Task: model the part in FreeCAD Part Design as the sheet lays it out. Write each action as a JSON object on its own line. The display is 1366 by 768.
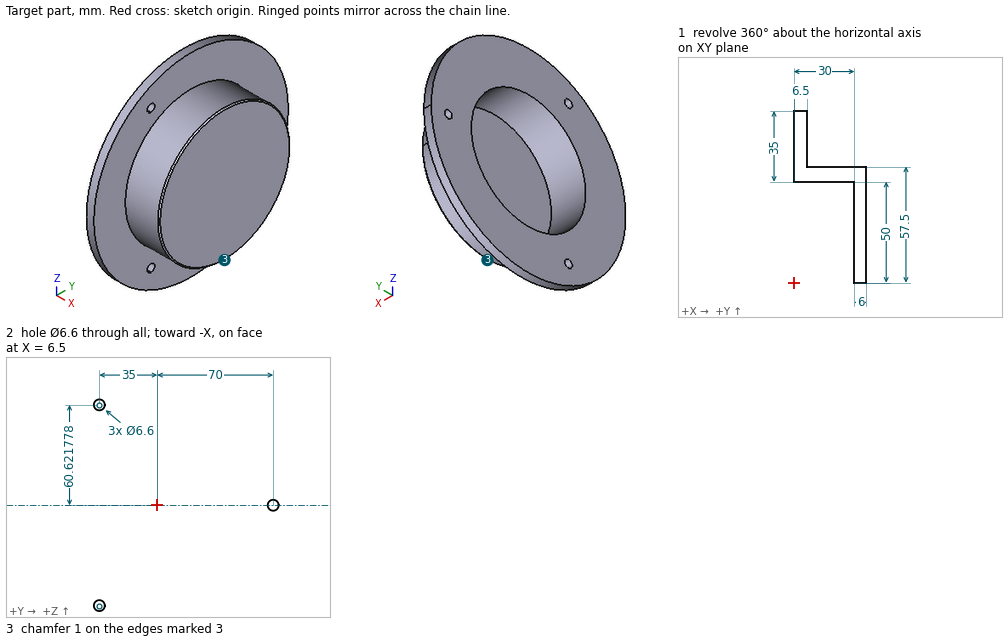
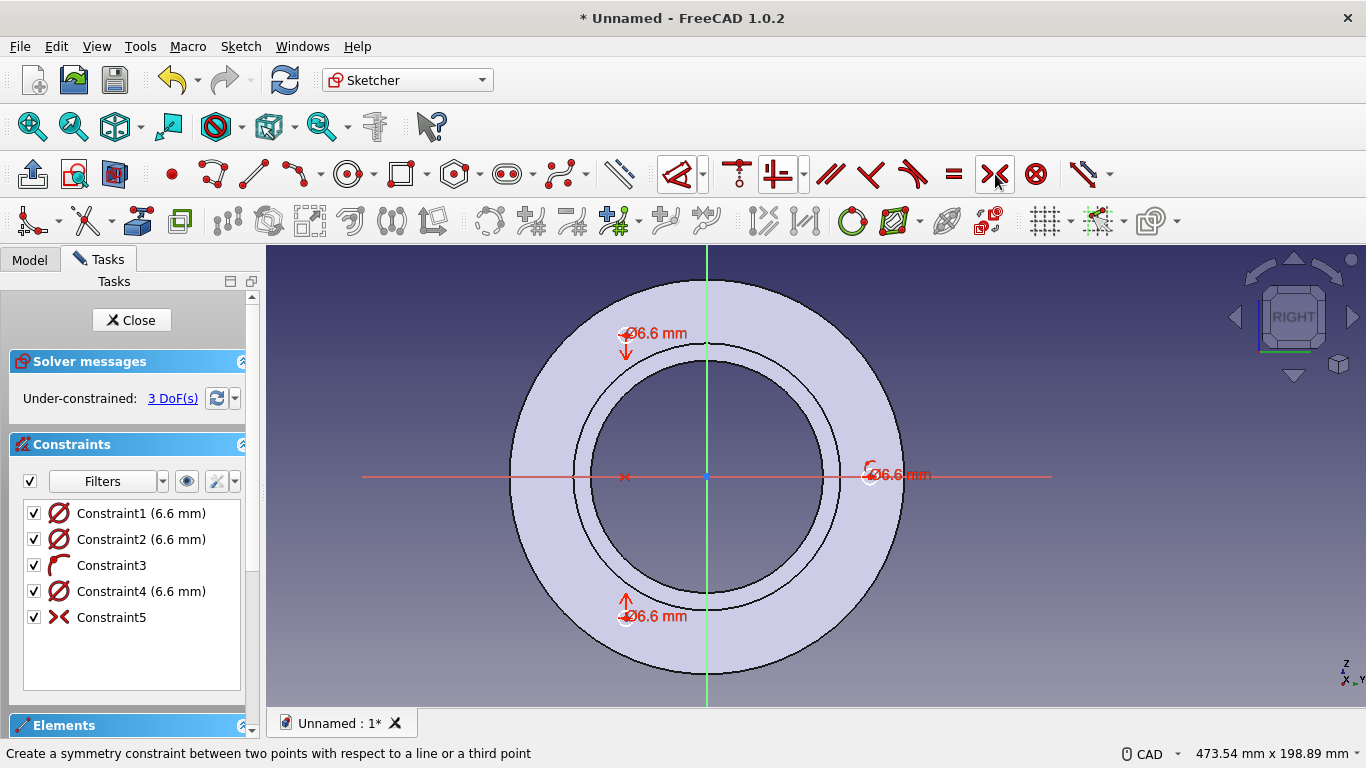
{"action": "left_click", "coordinate": [626, 335]}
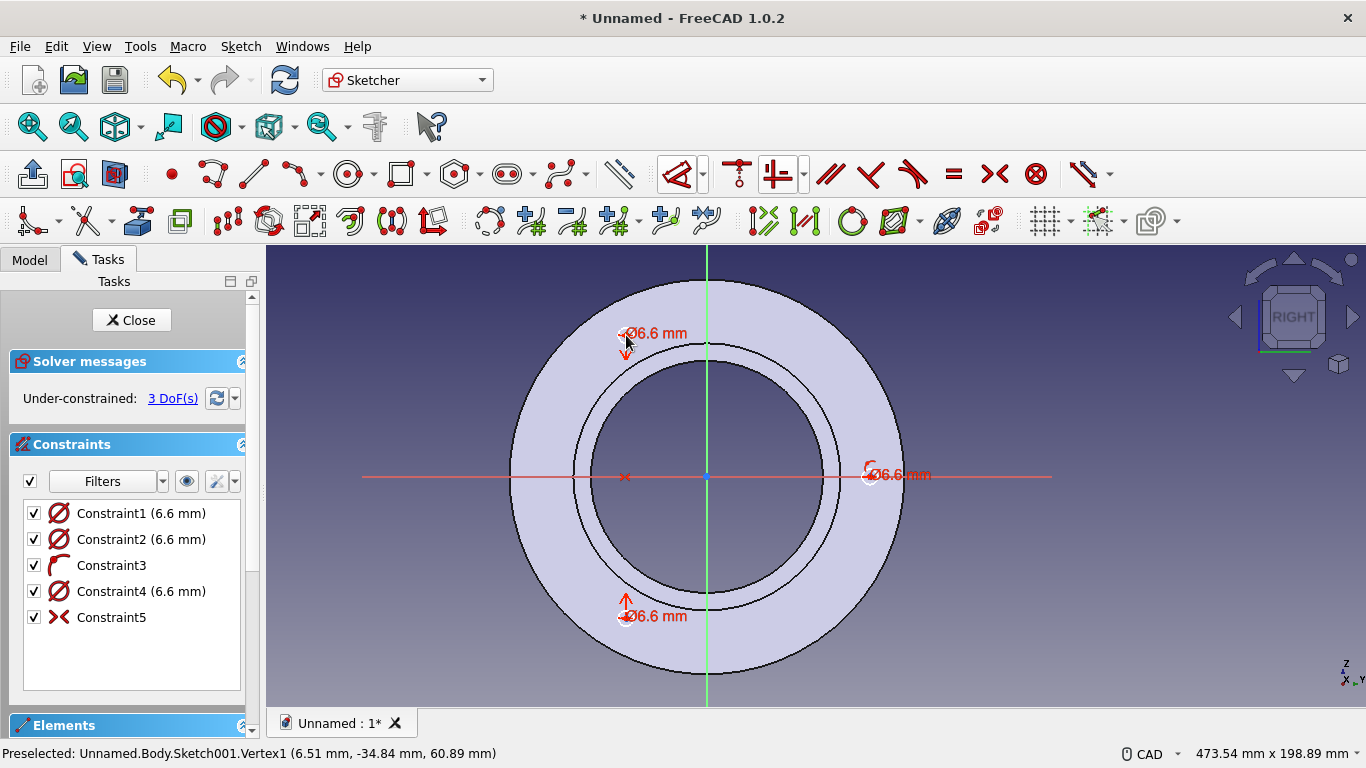
{"action": "left_click", "coordinate": [702, 174]}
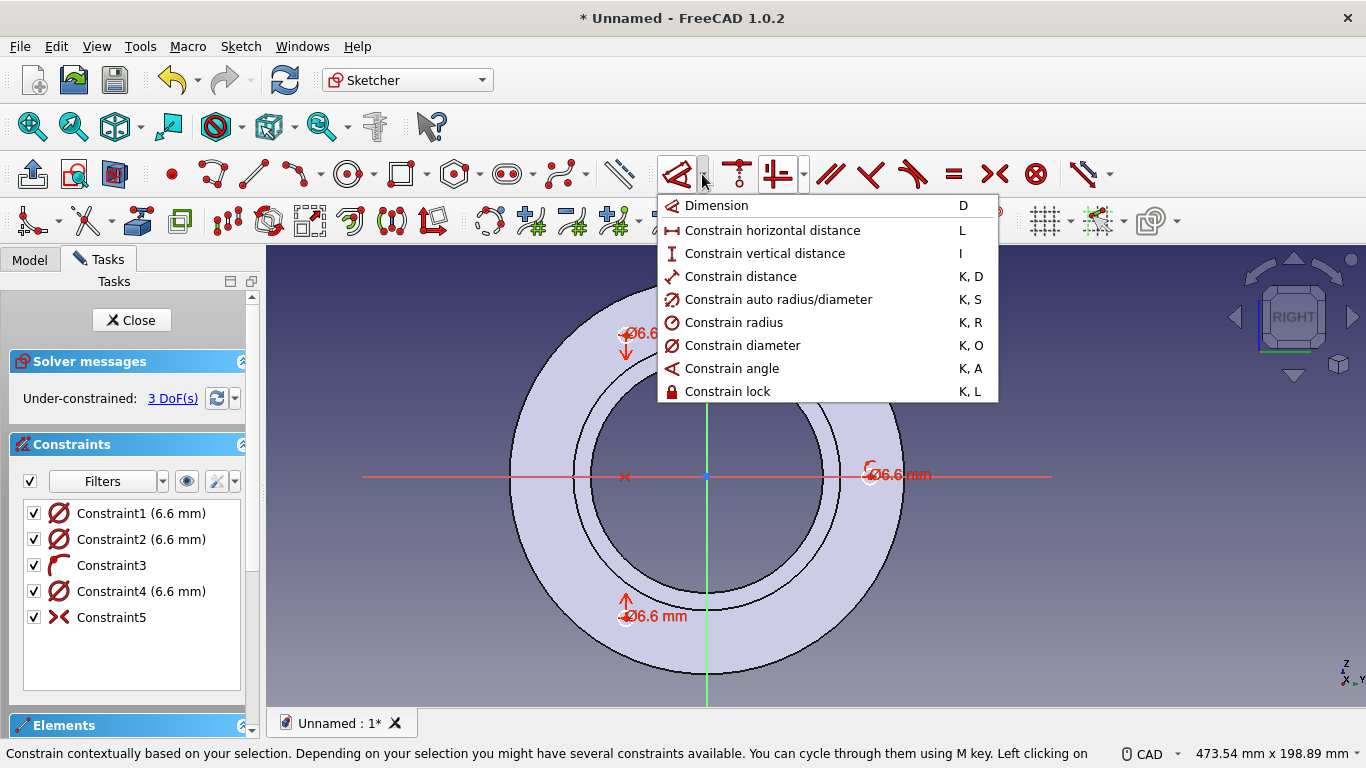
{"action": "left_click", "coordinate": [828, 230]}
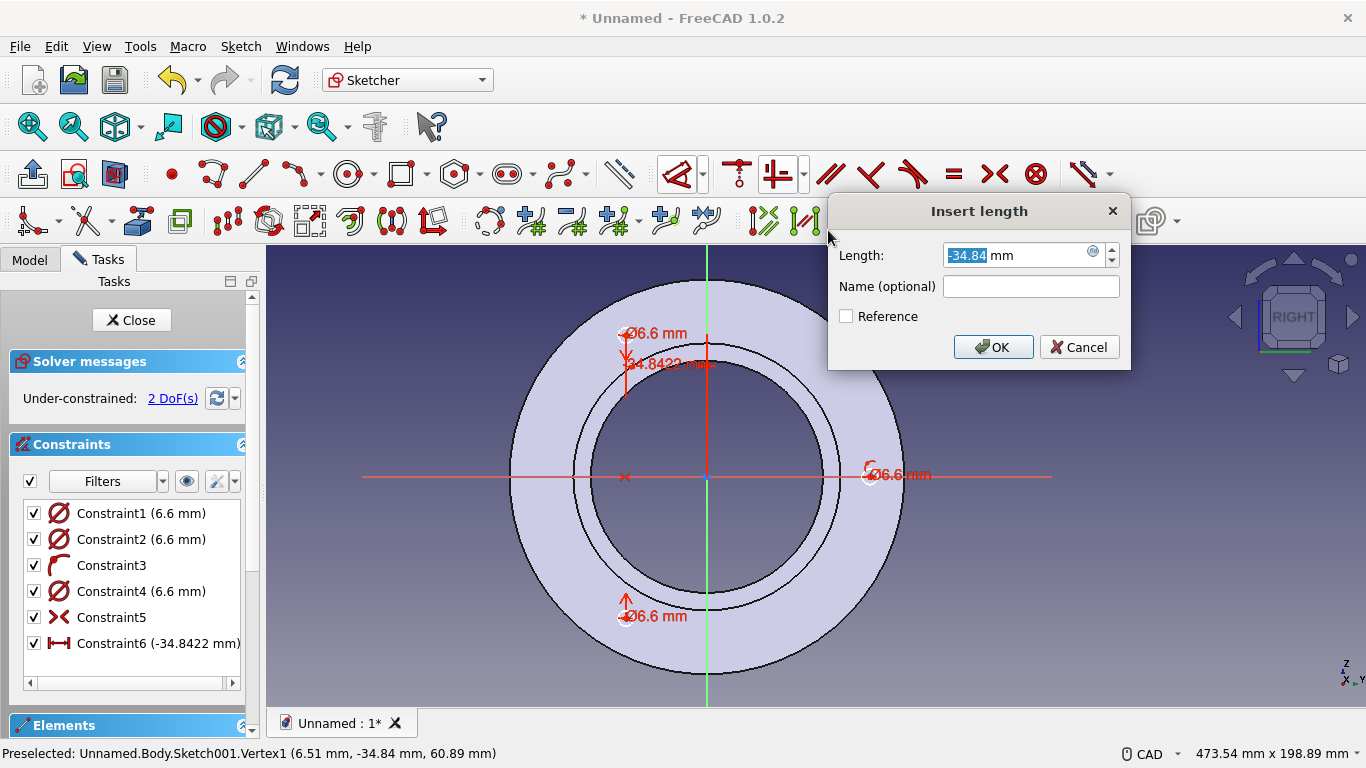
{"action": "type", "text": "-35"}
{"action": "key", "text": "Return"}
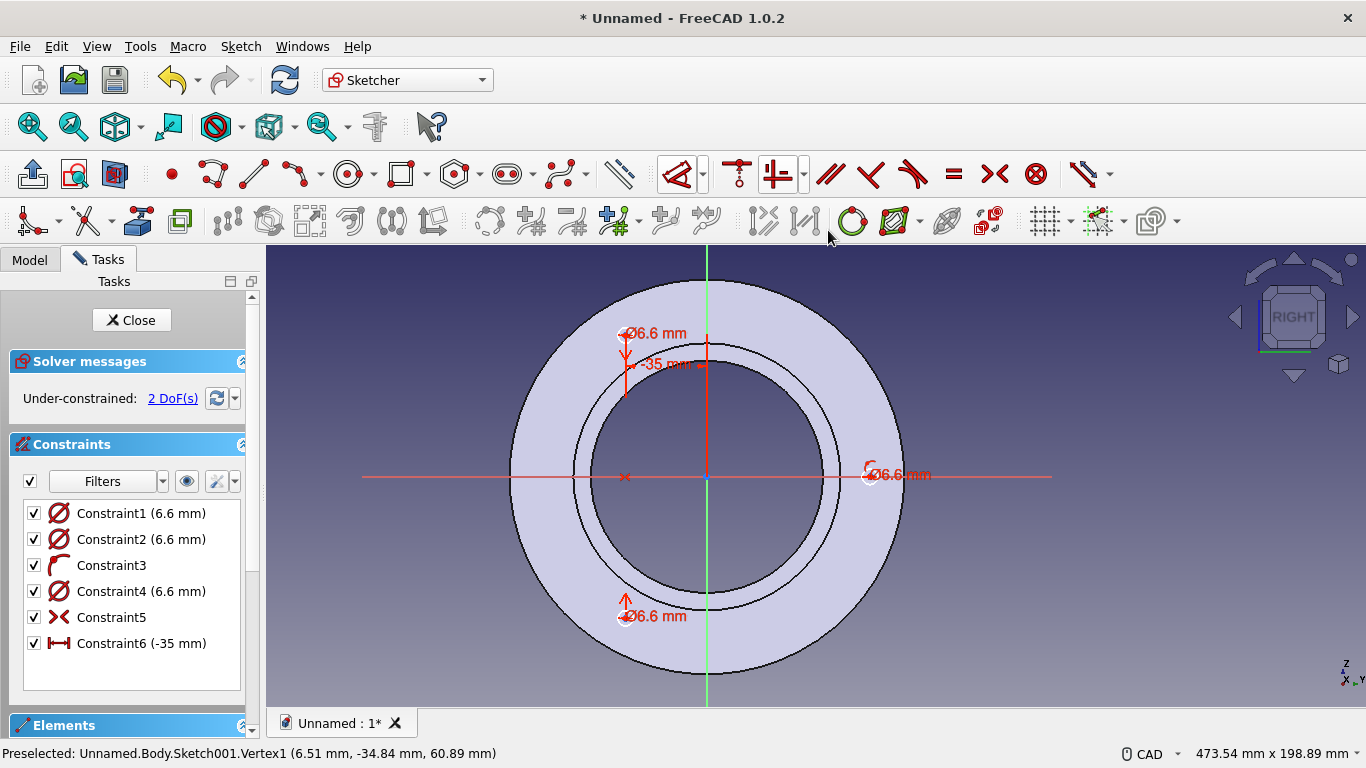
{"action": "left_click", "coordinate": [870, 477]}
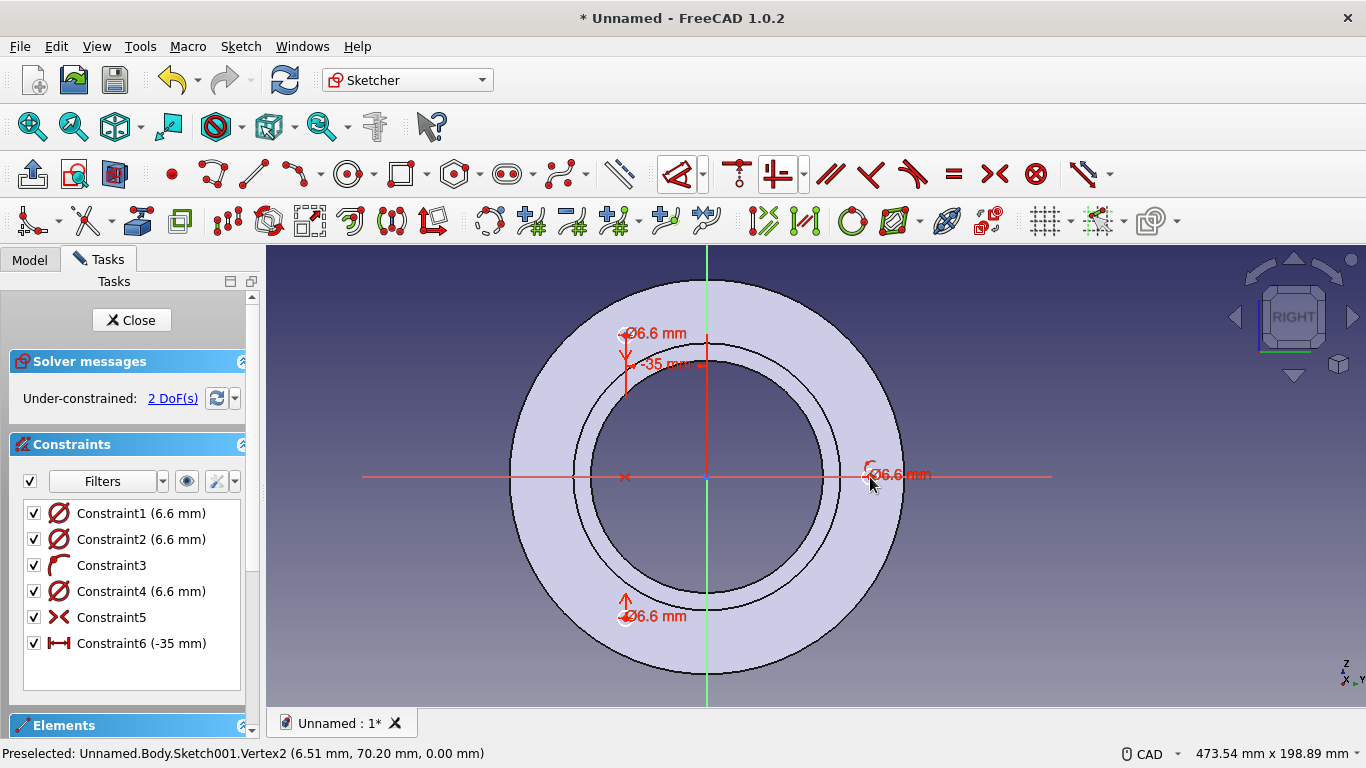
{"action": "key", "text": "l"}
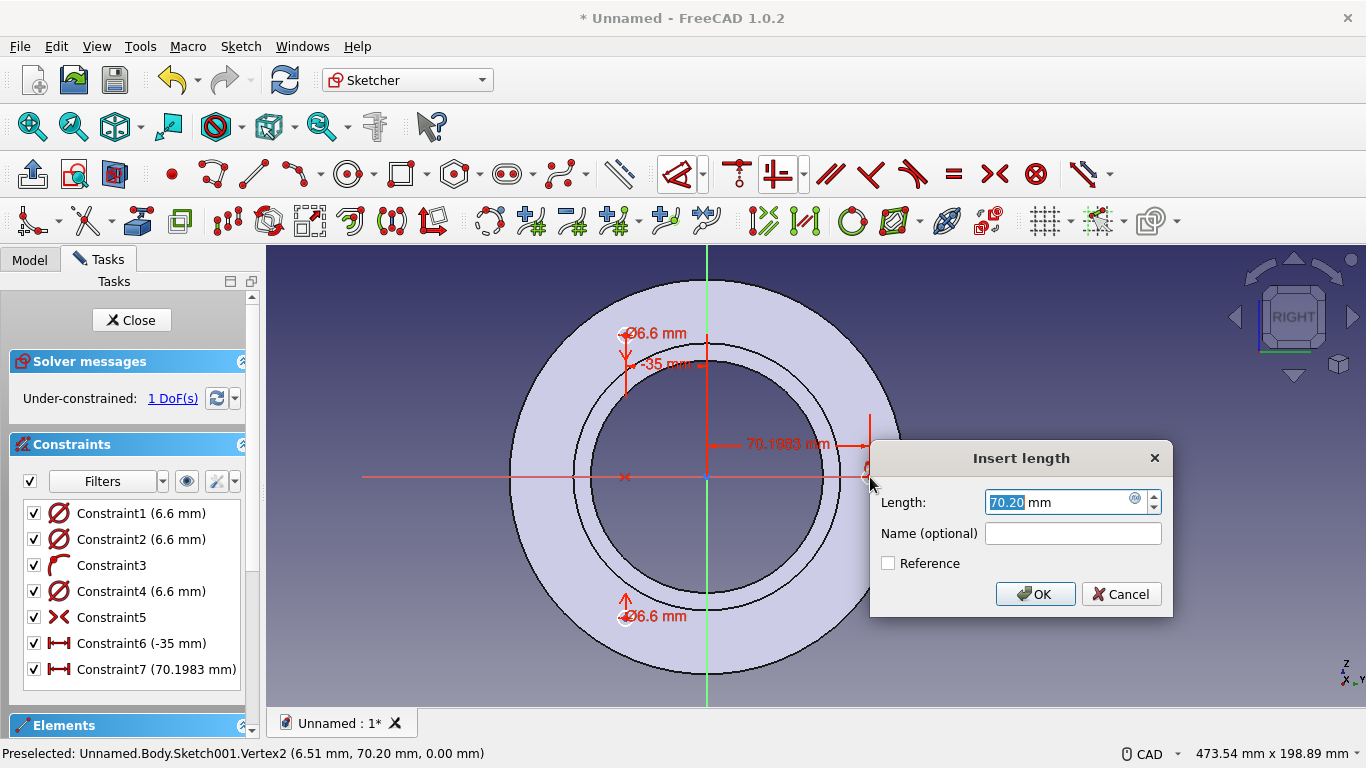
{"action": "type", "text": "70"}
{"action": "key", "text": "Return"}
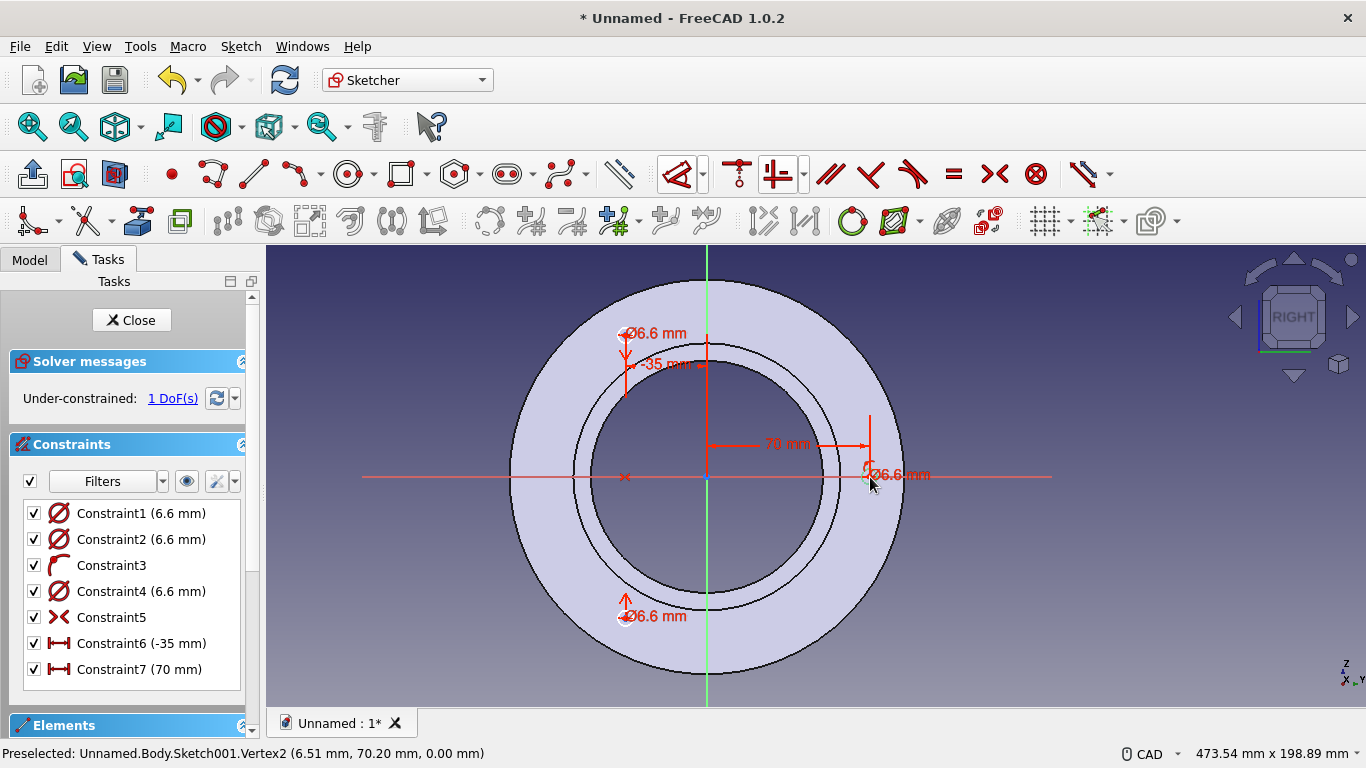
{"action": "left_click", "coordinate": [626, 335]}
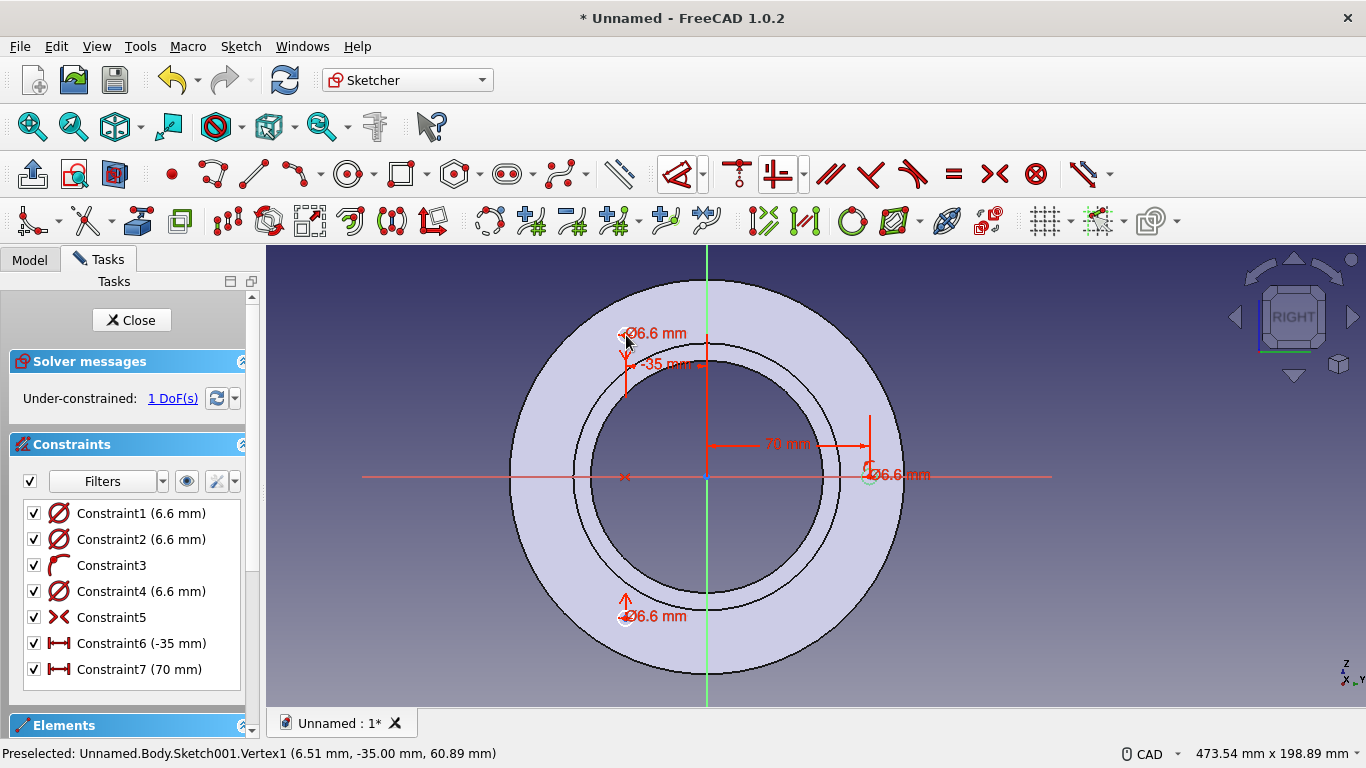
{"action": "key", "text": "i"}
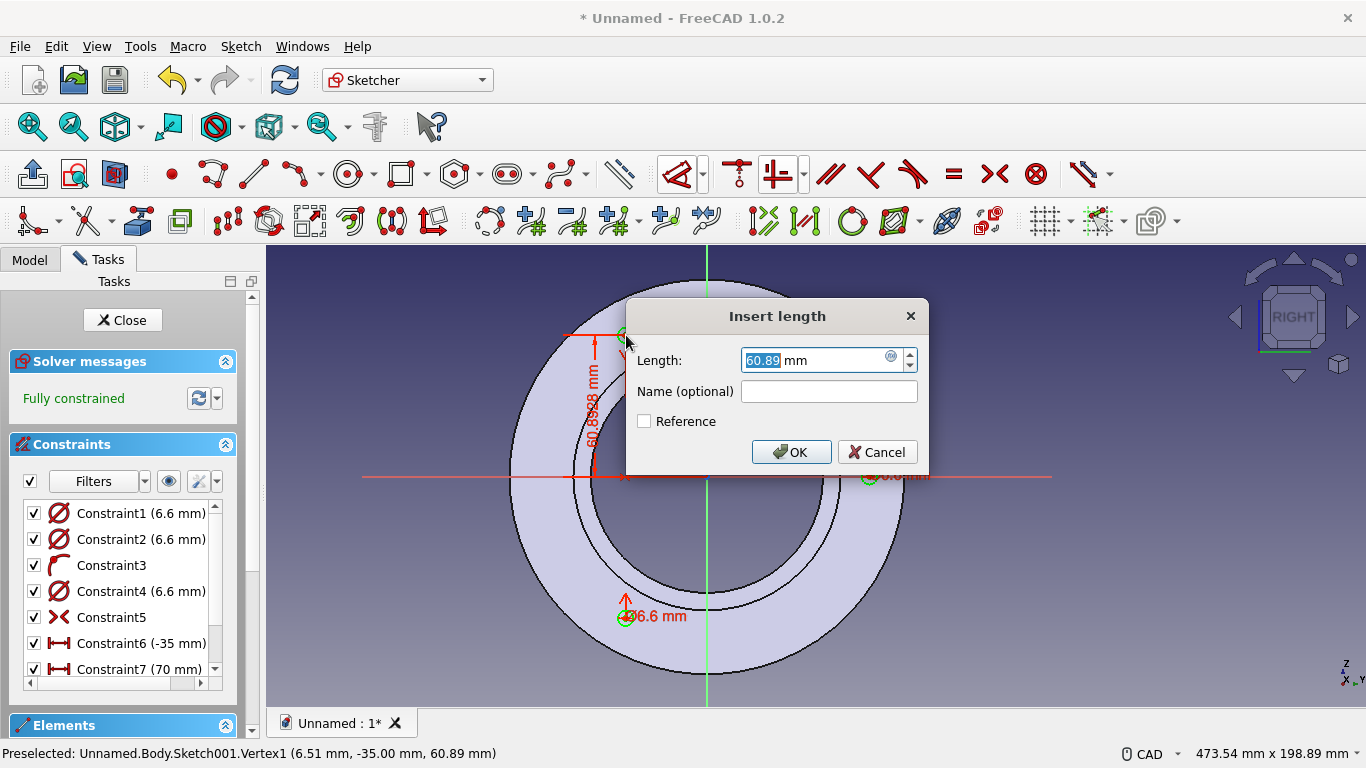
{"action": "type", "text": "60.621778"}
{"action": "key", "text": "Return"}